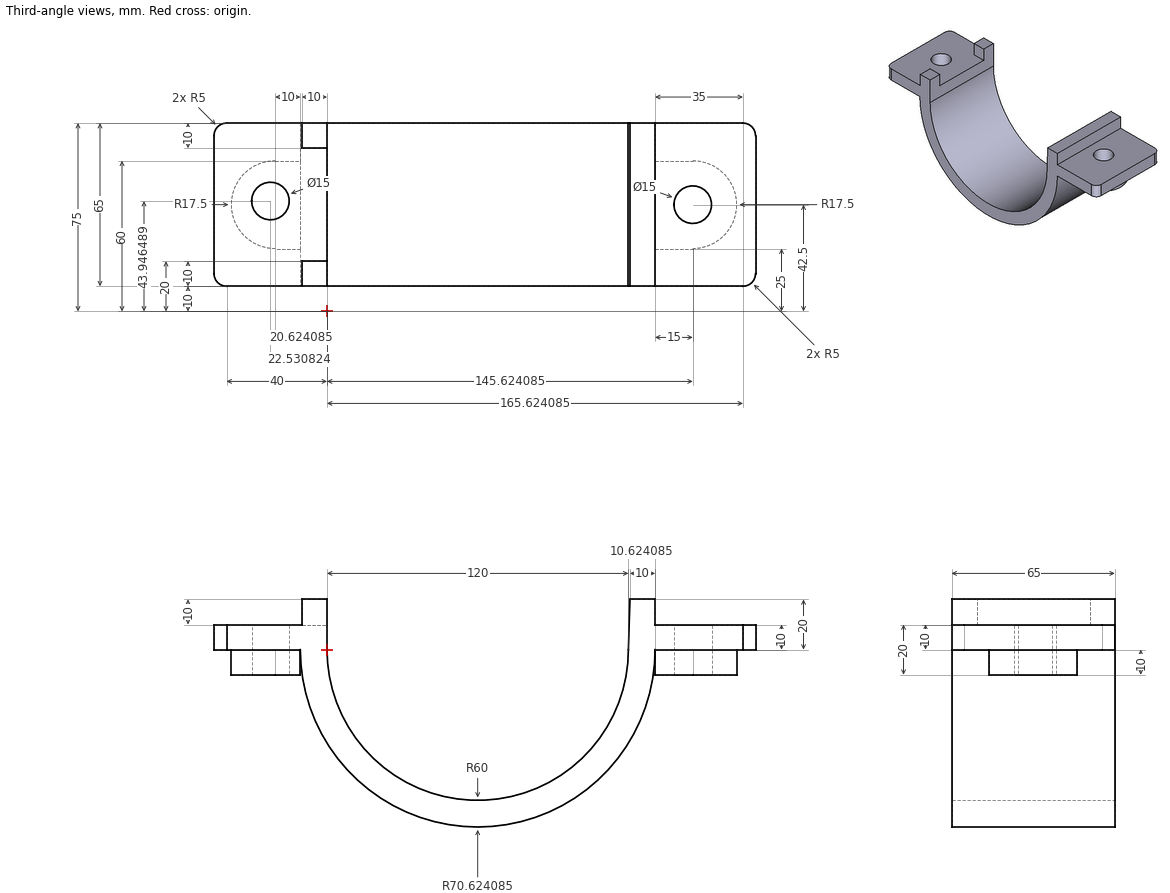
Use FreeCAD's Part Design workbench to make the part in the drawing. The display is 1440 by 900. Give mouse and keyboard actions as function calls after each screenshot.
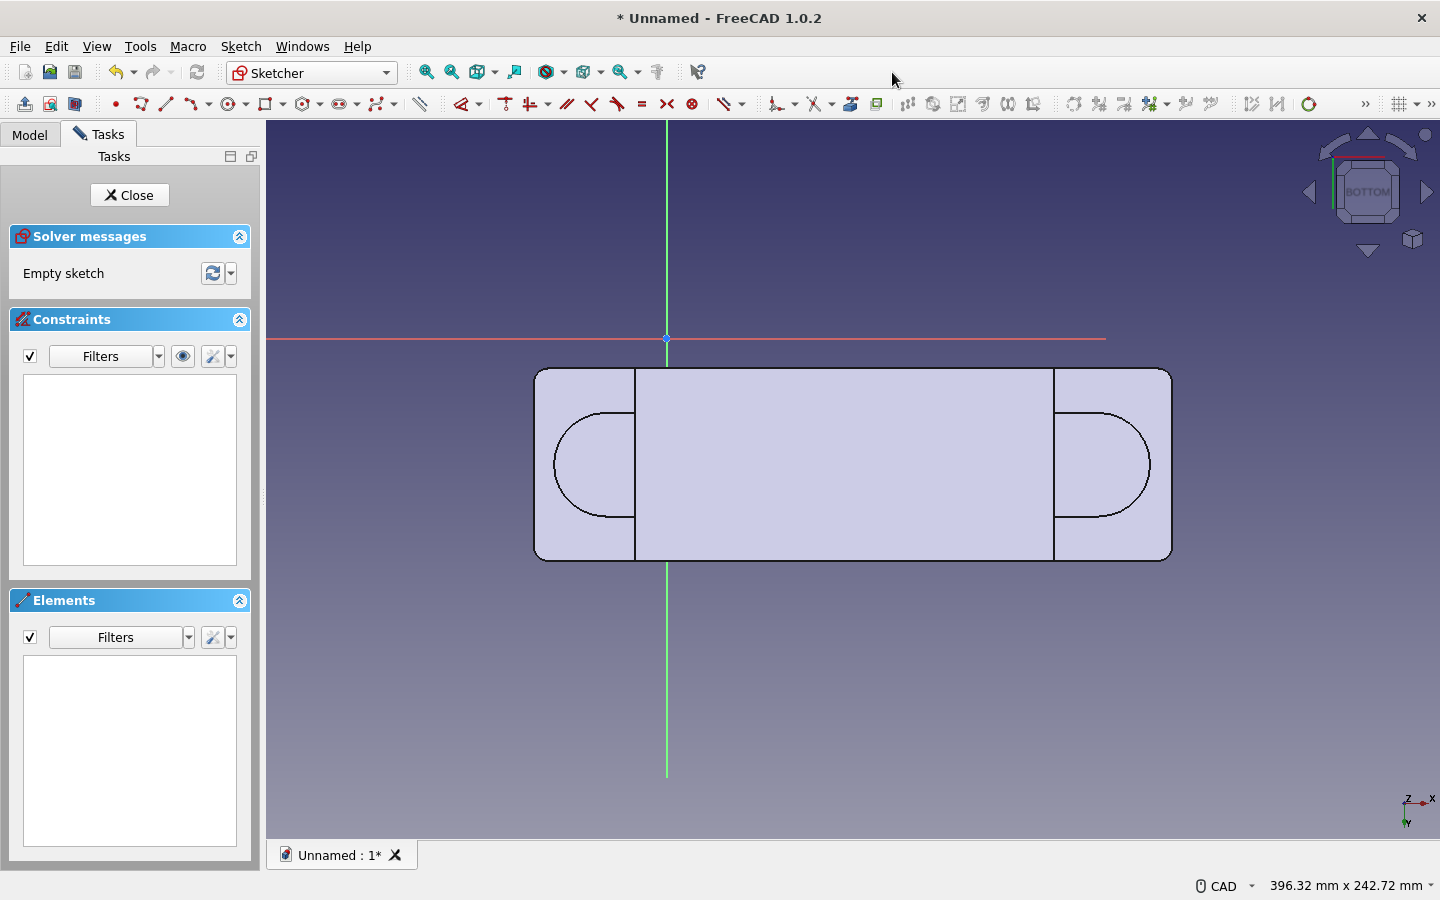
scroll(1130, 463, up, 12)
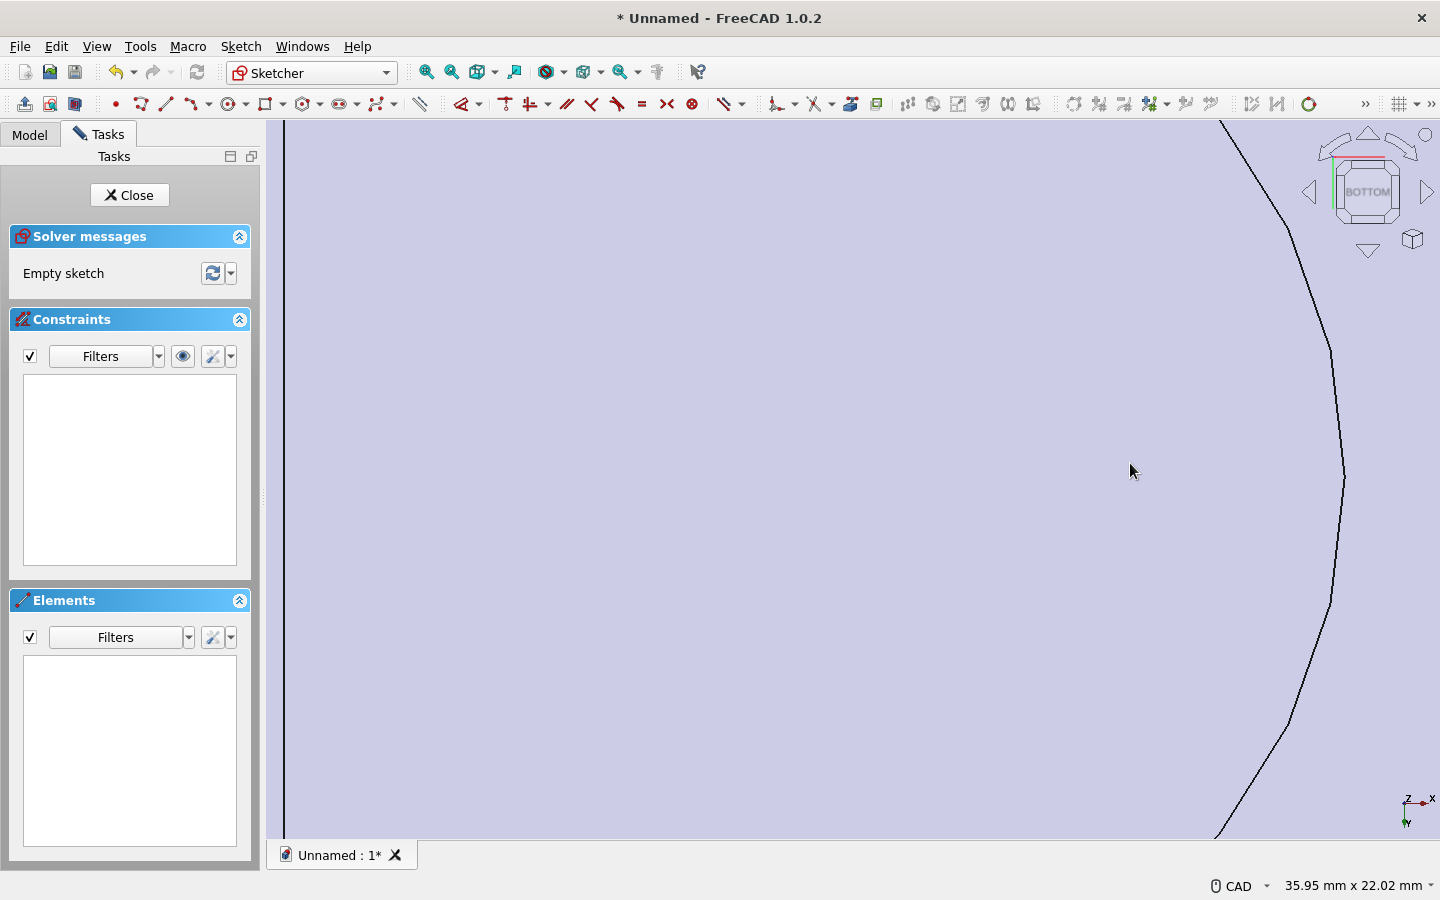
key(g)
key(c)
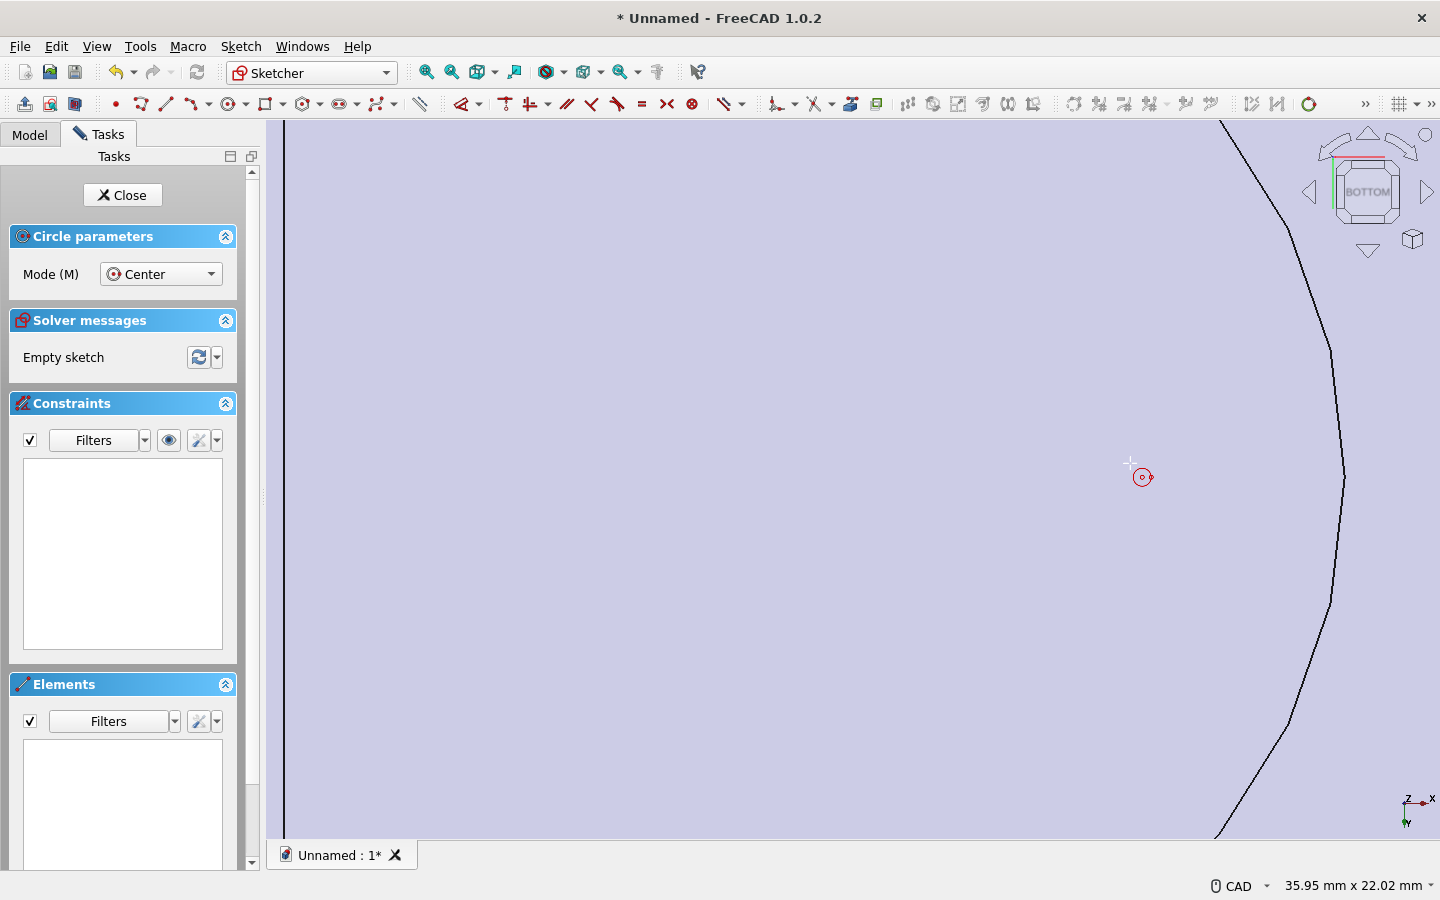
click(773, 477)
move(946, 304)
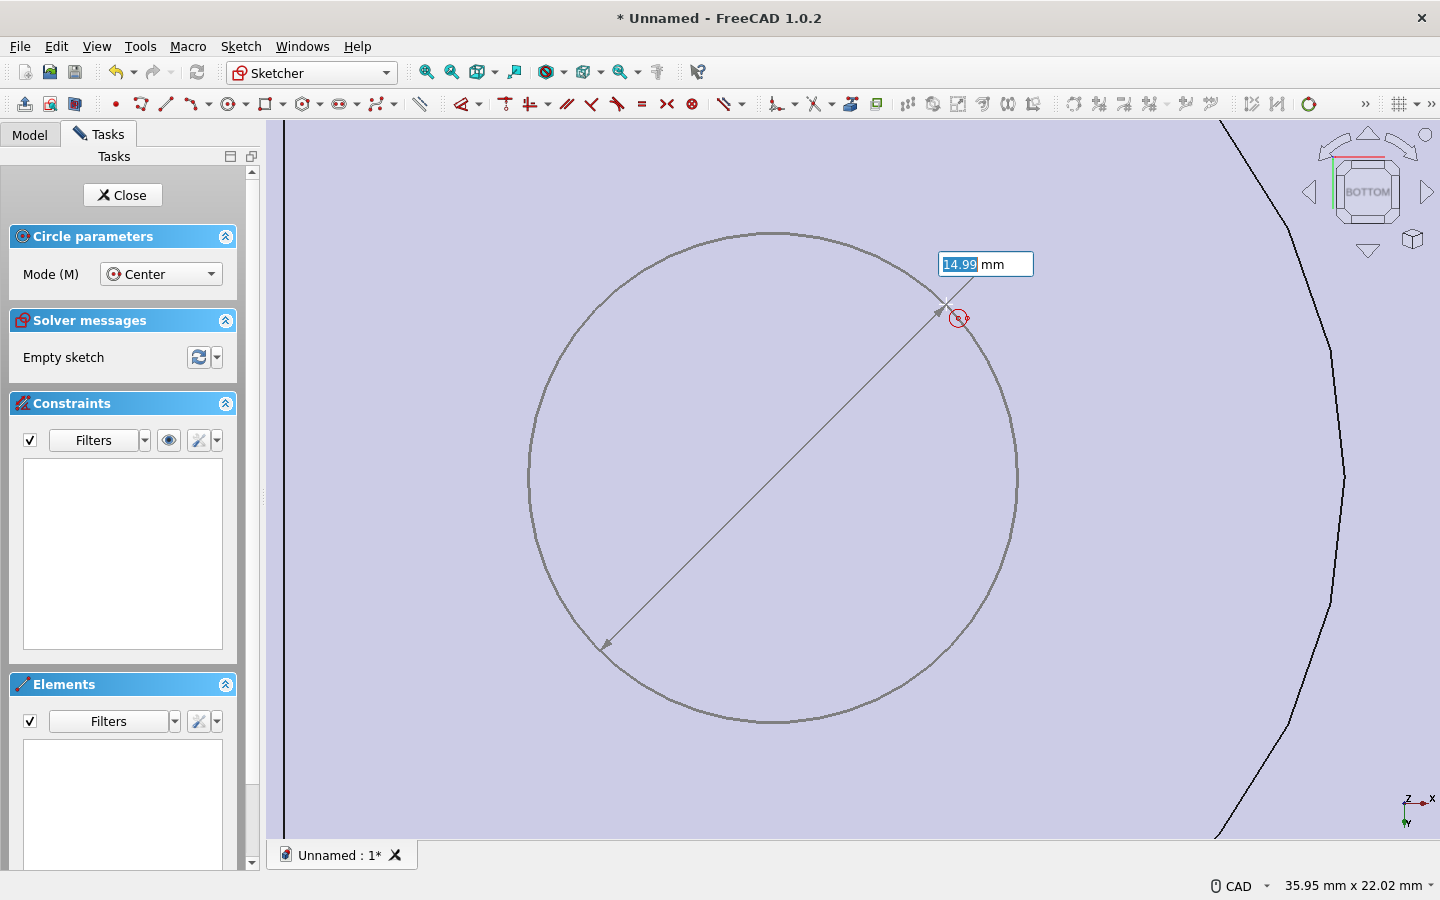
text(15)
key(Return)
key(Escape)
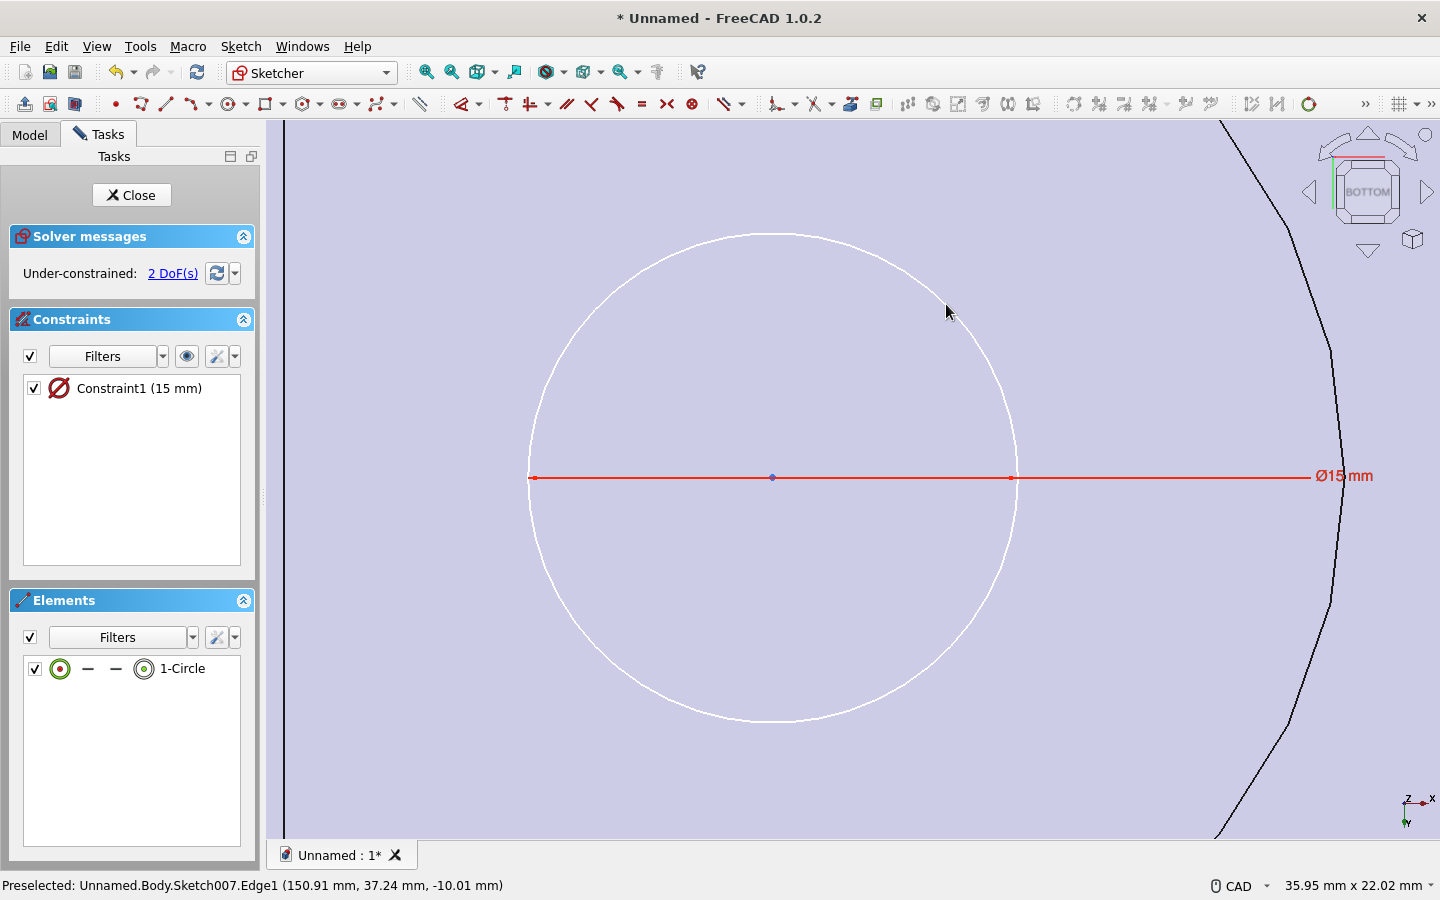
click(460, 104)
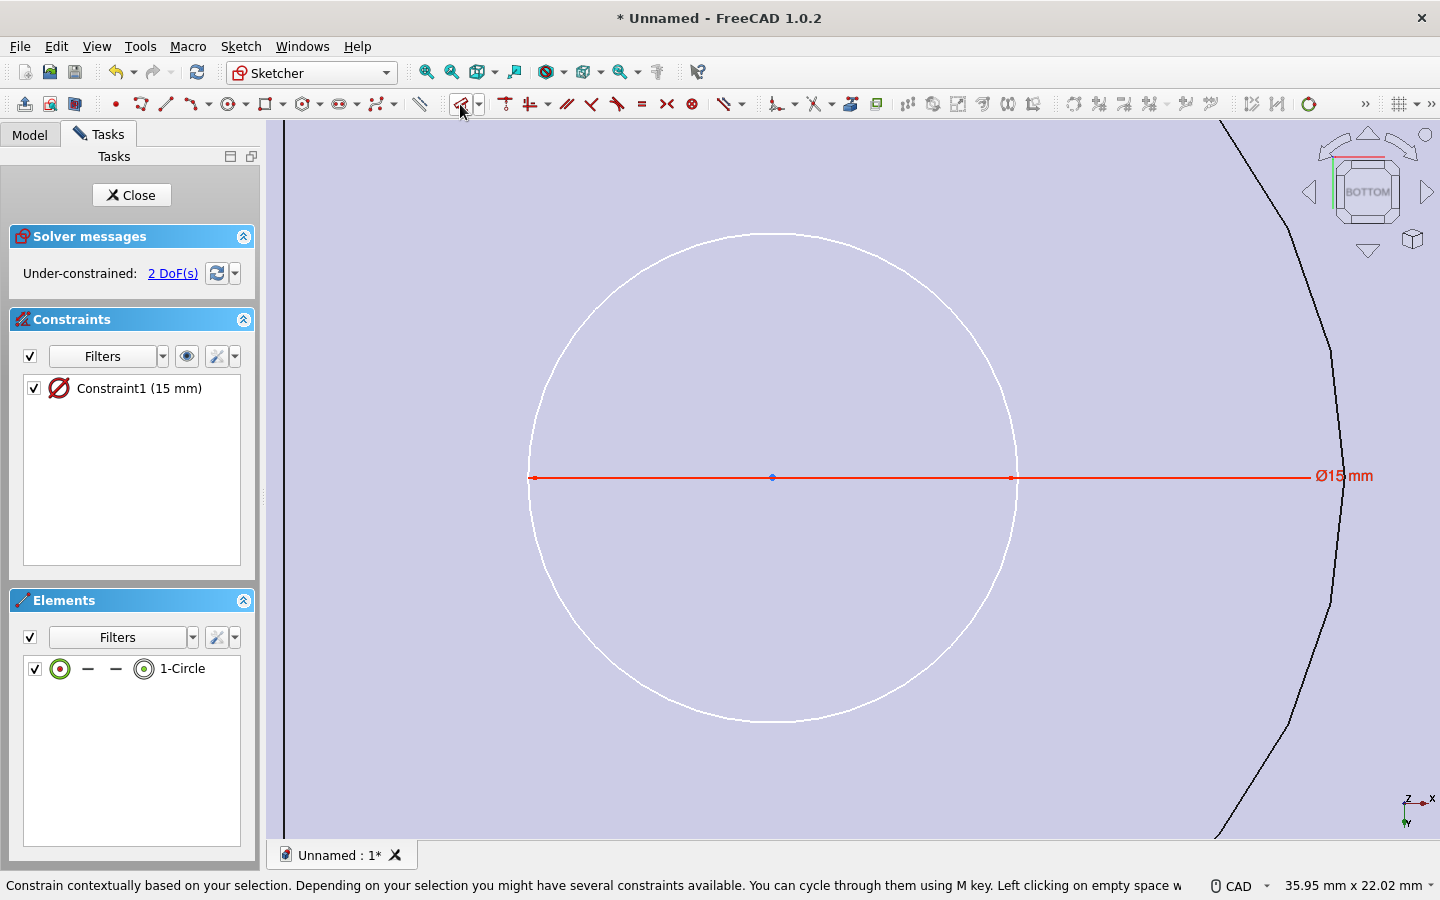
click(773, 478)
click(807, 313)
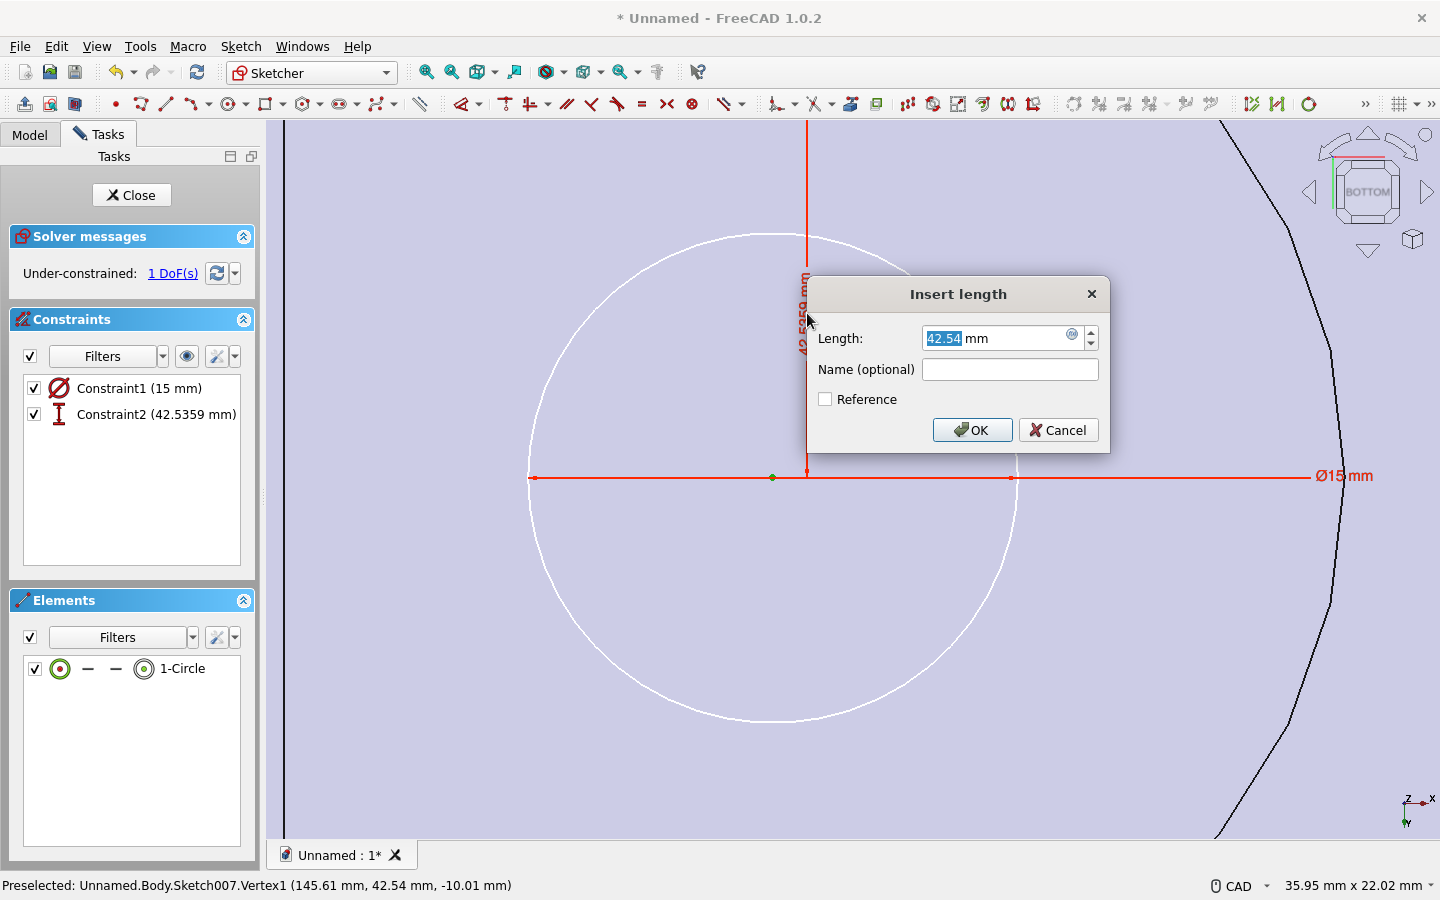
text(42.5)
key(Return)